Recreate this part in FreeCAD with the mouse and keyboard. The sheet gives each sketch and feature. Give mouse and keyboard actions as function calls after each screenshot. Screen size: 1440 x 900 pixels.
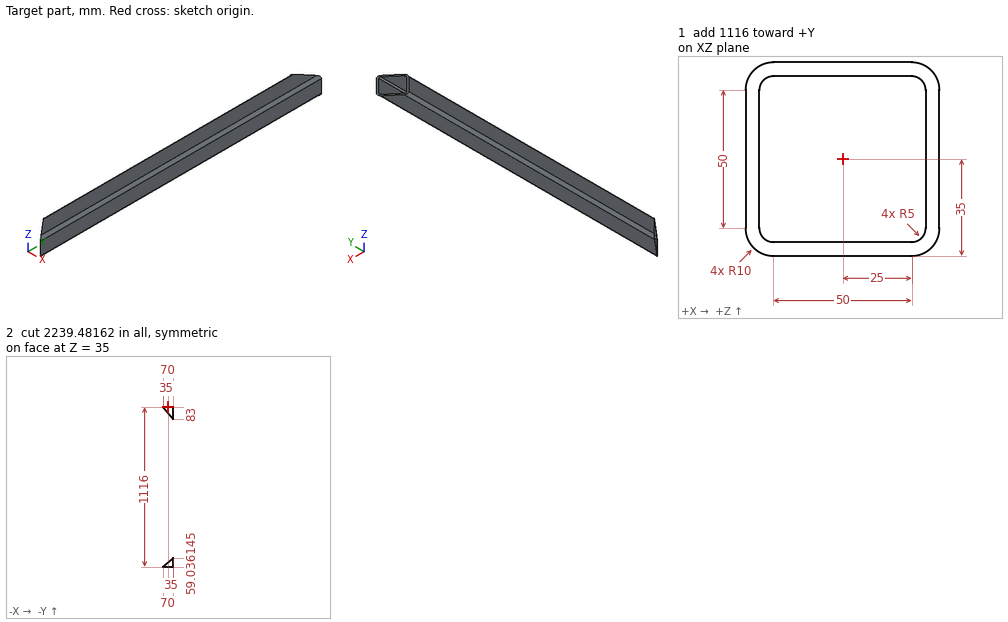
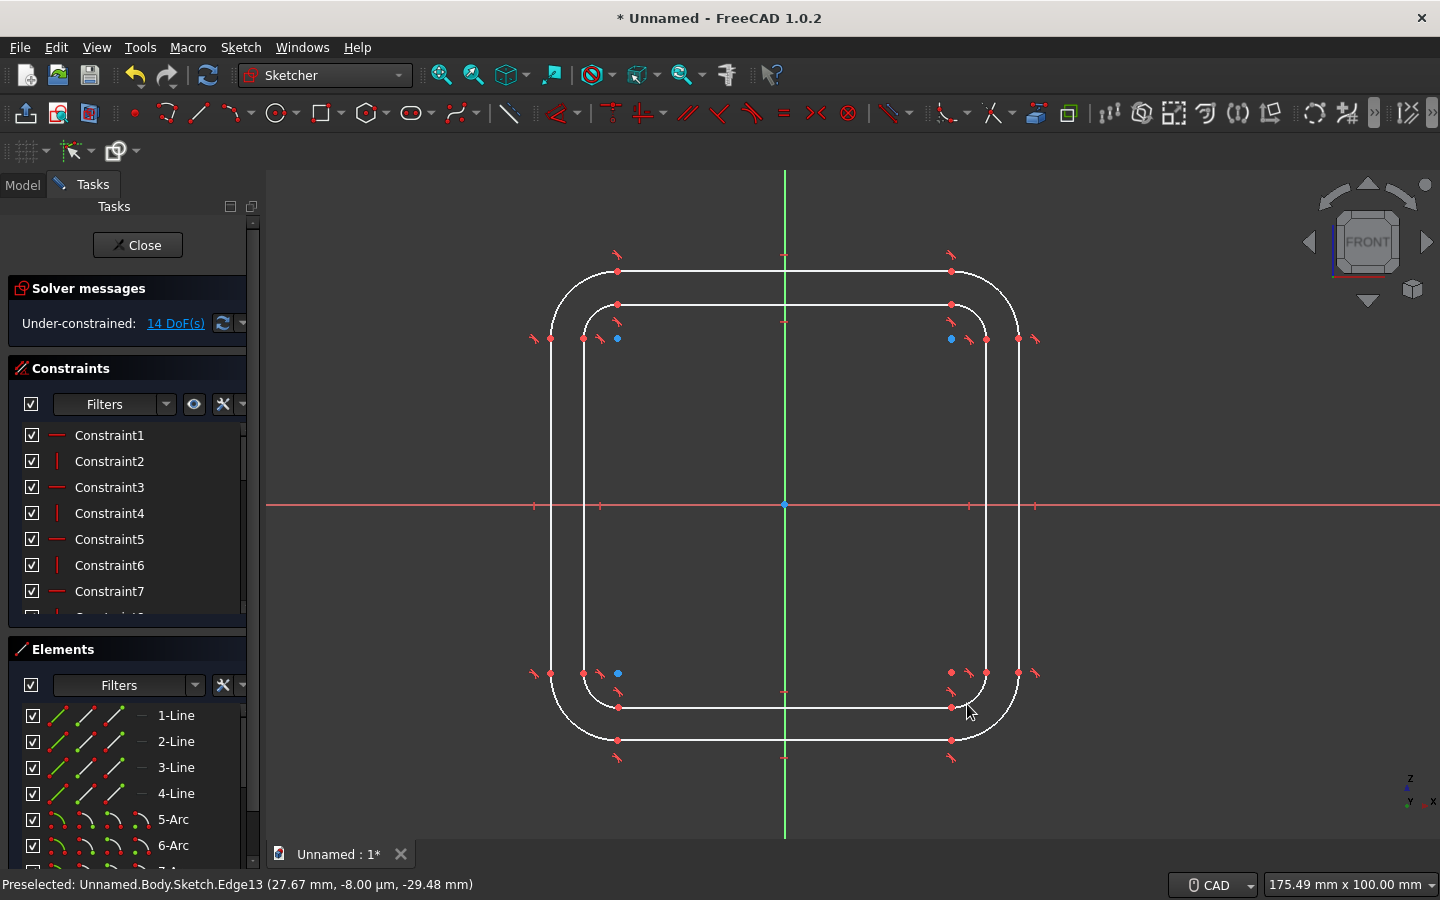
click(1012, 308)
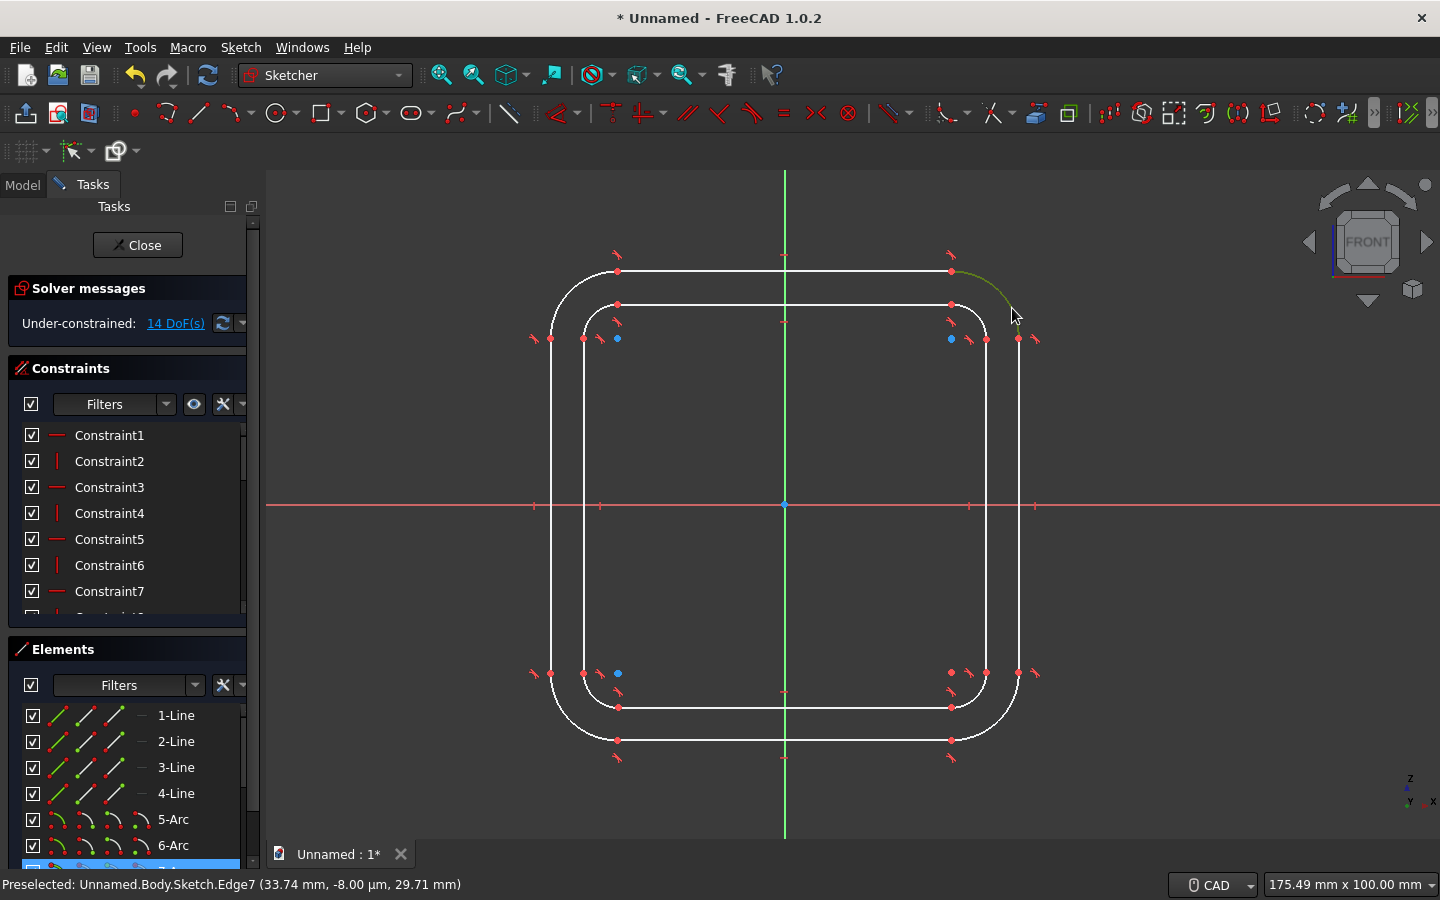
click(983, 323)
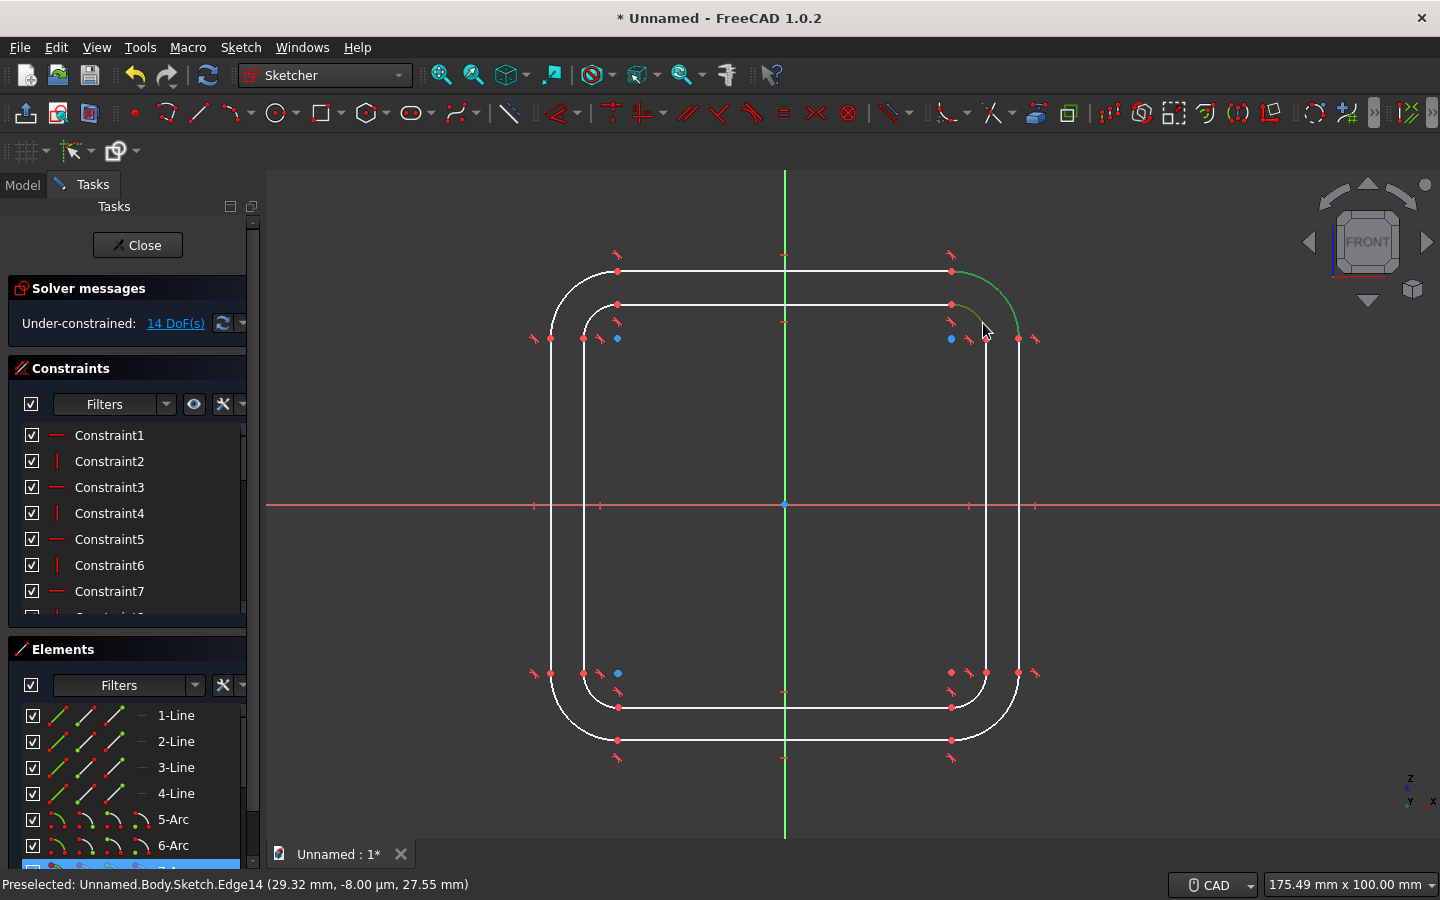
click(612, 114)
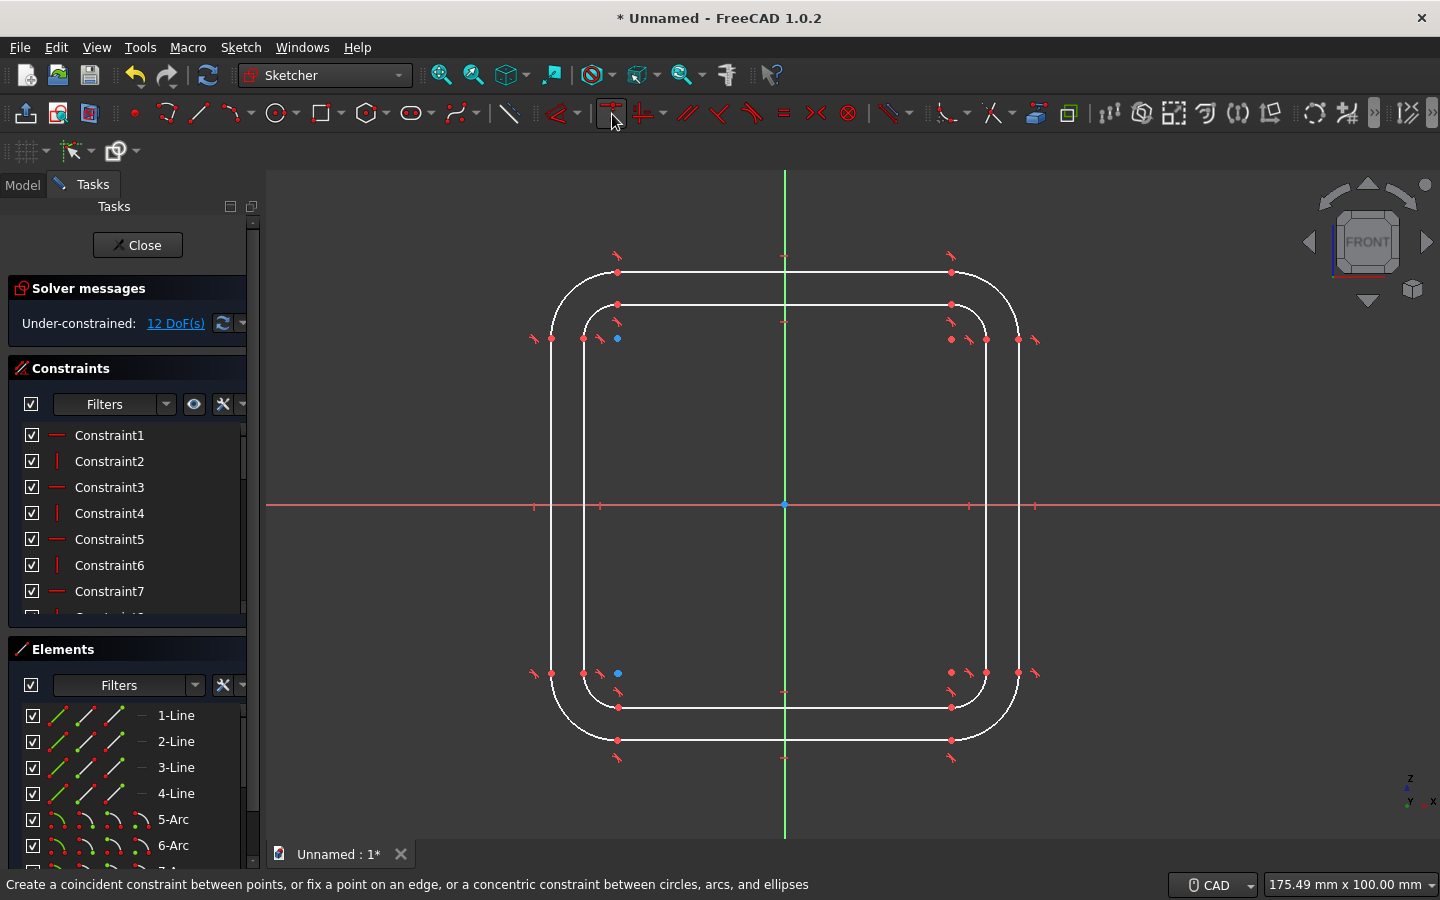
click(587, 279)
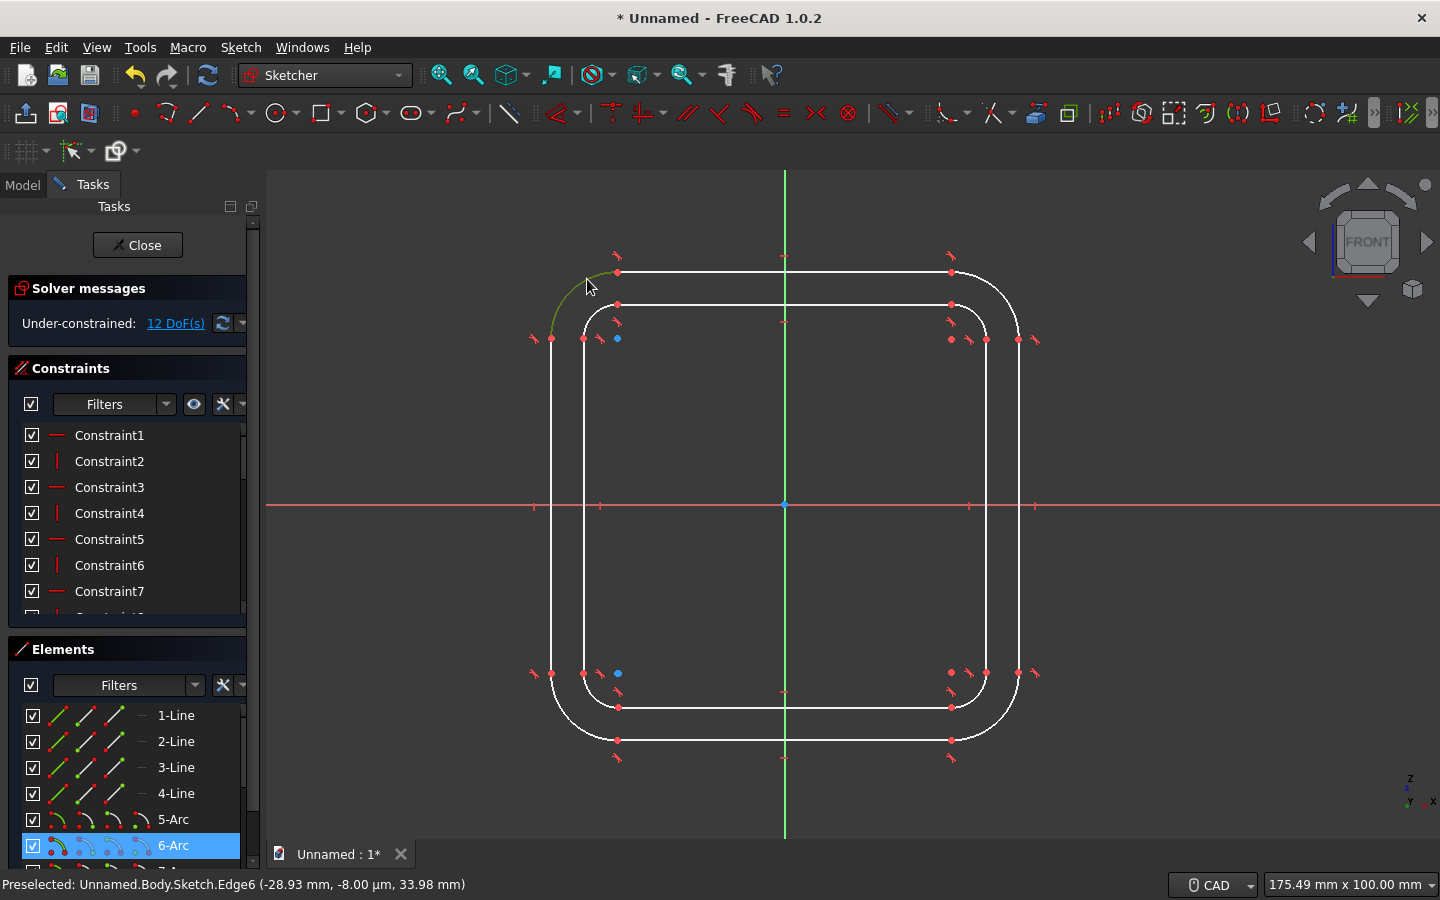
click(602, 308)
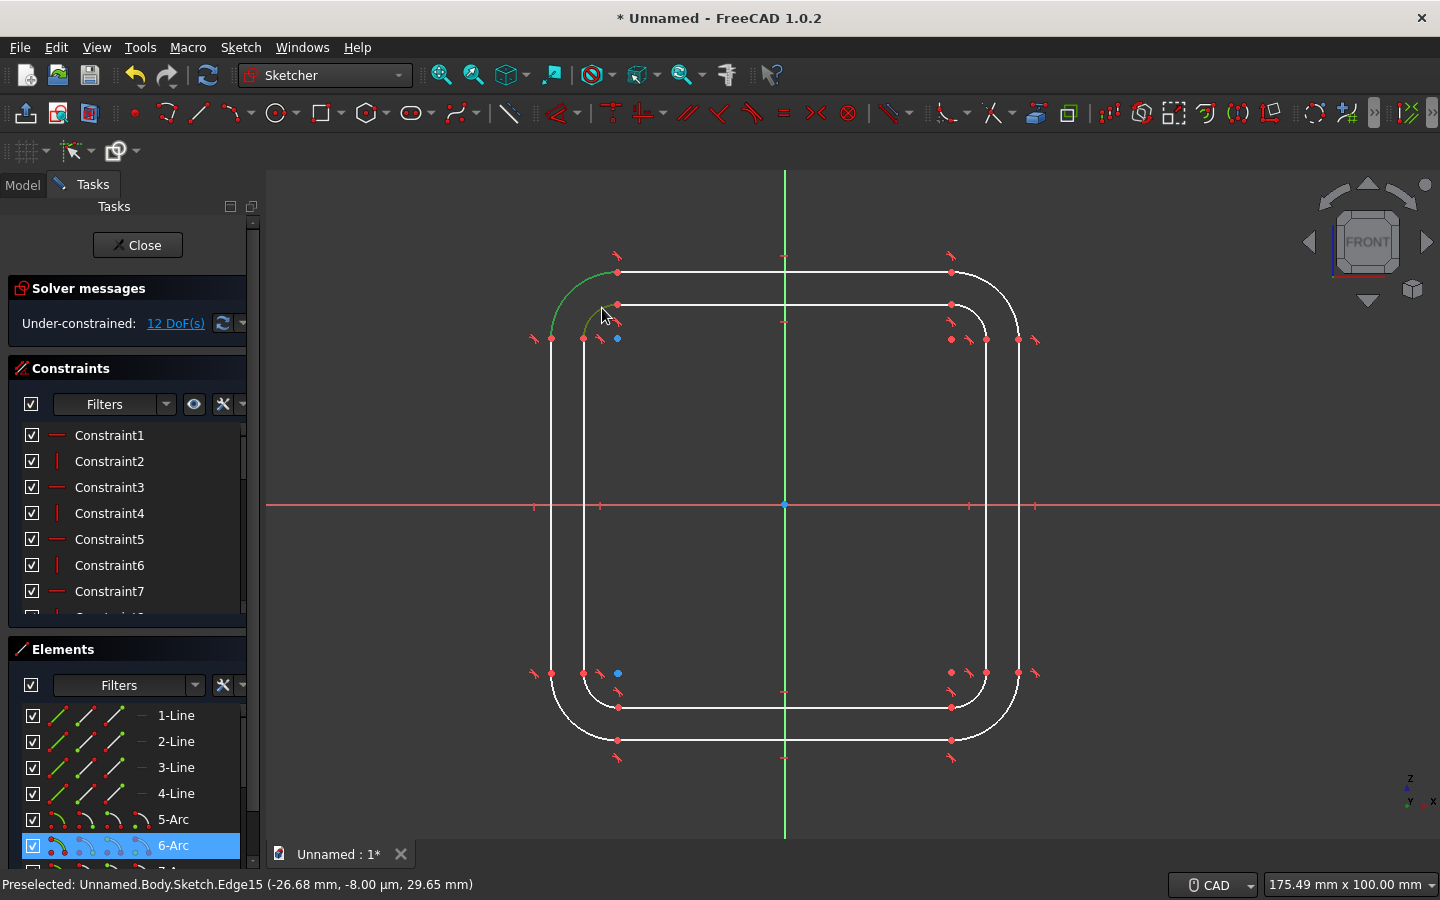
key(c)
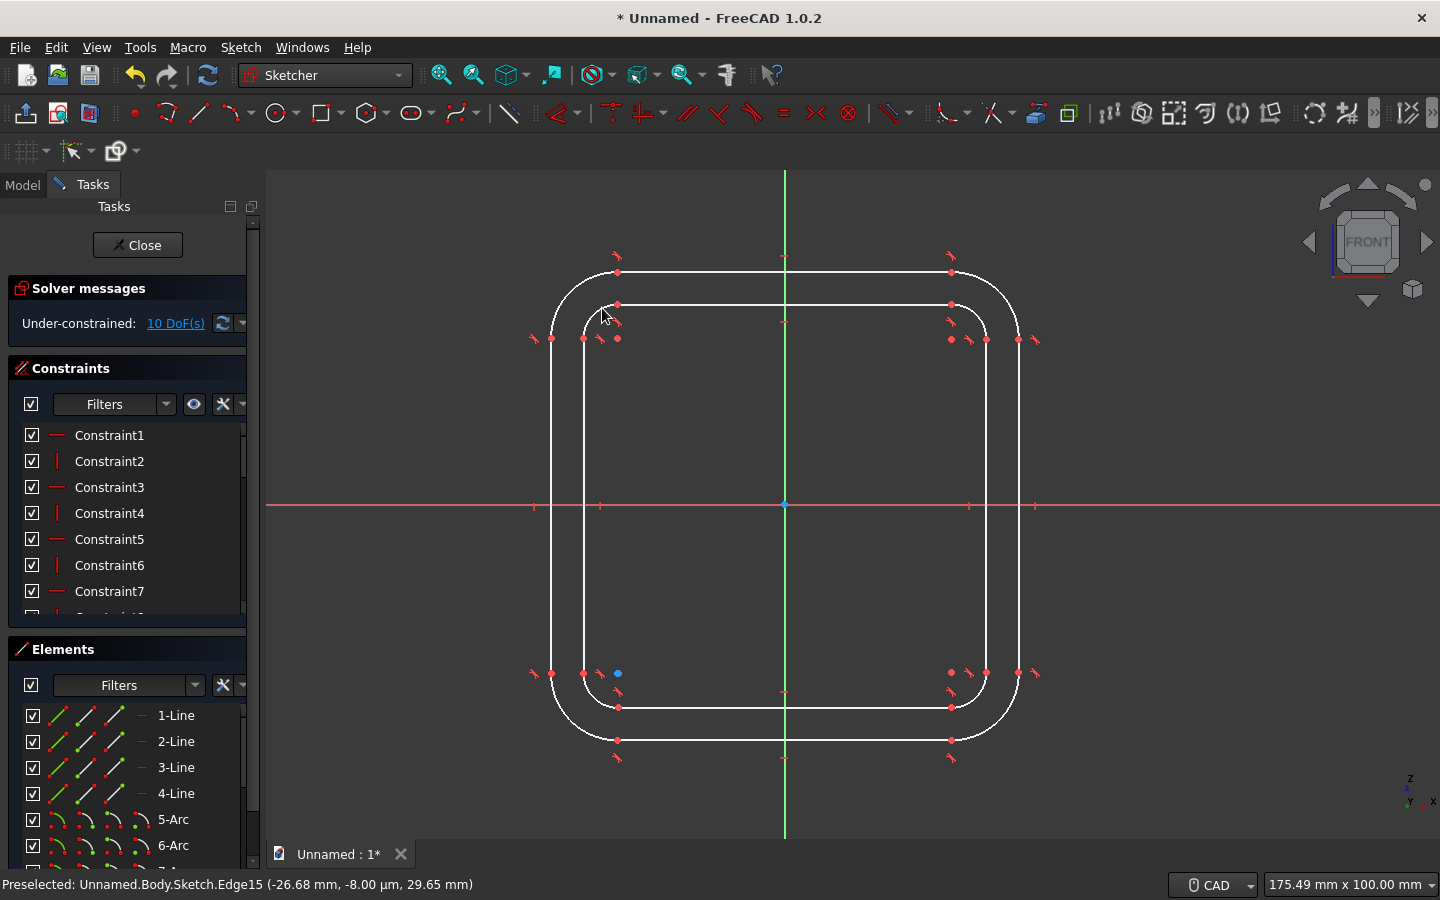
click(558, 704)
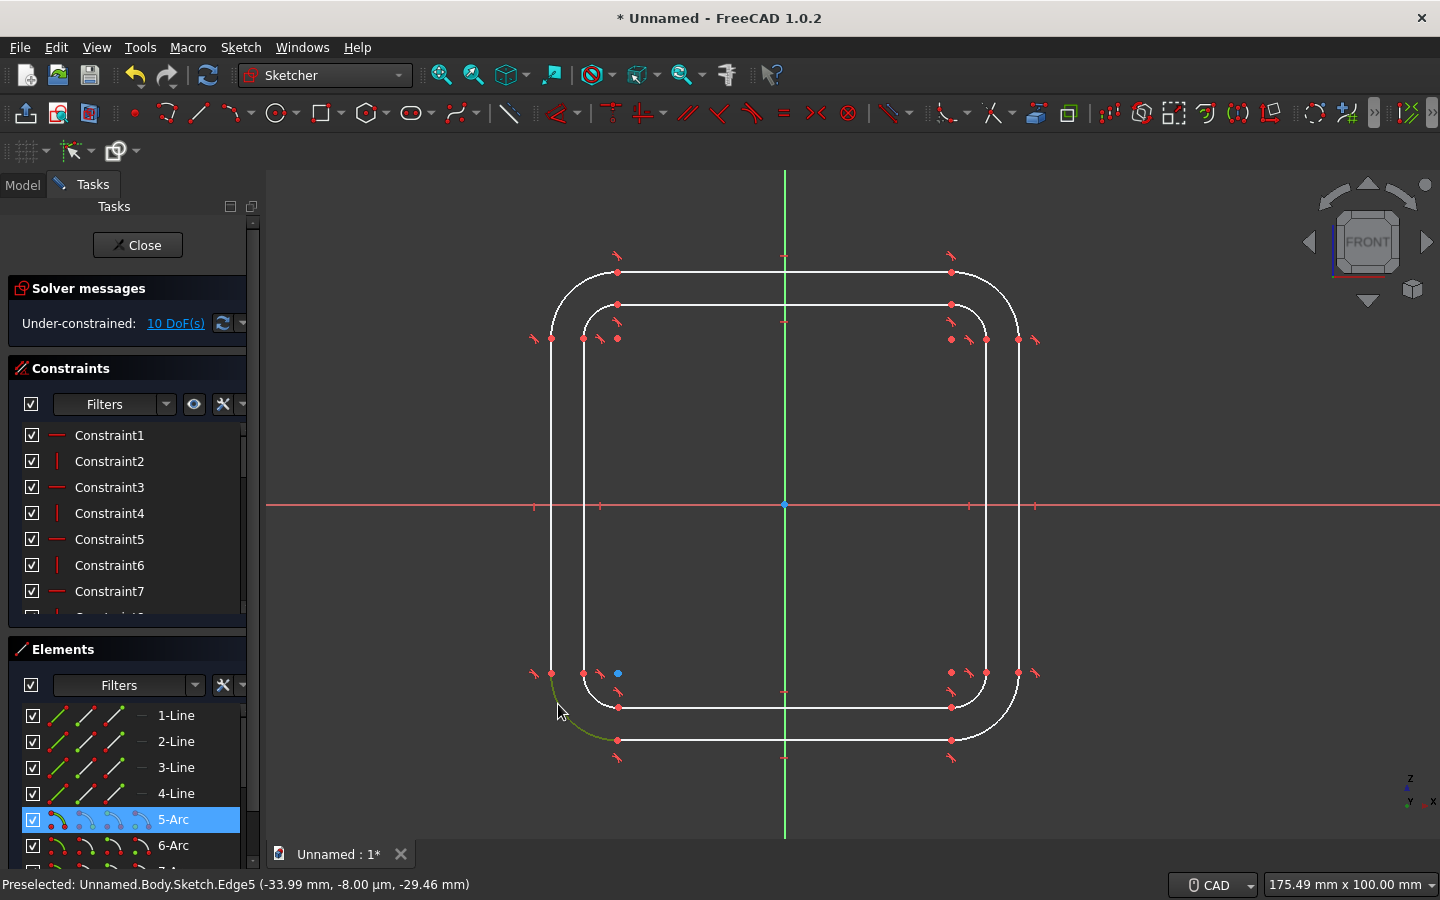
click(587, 279)